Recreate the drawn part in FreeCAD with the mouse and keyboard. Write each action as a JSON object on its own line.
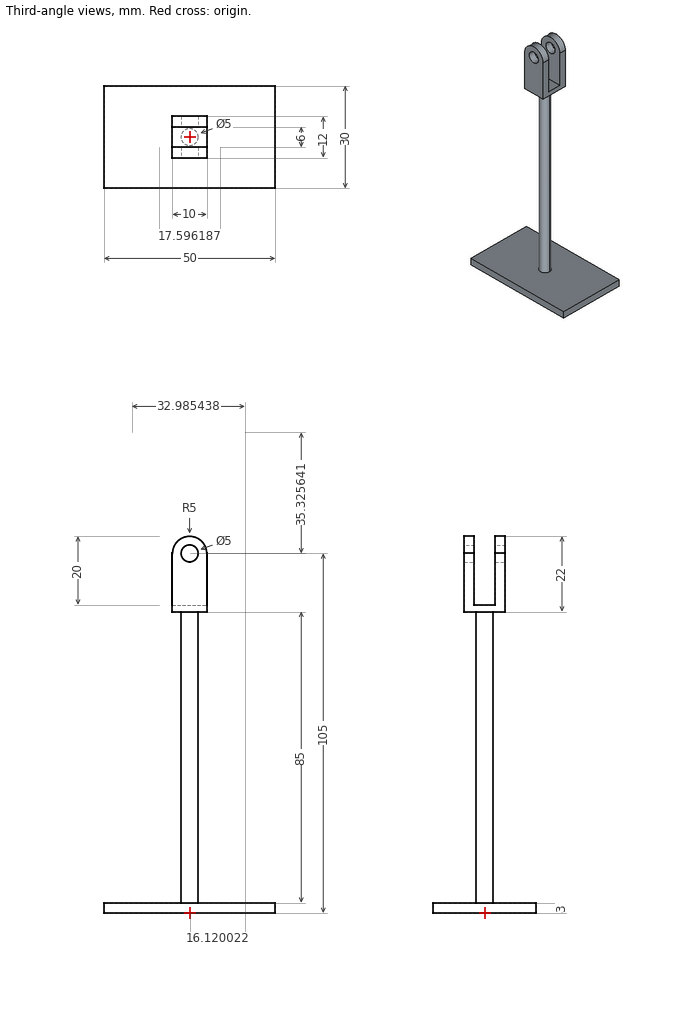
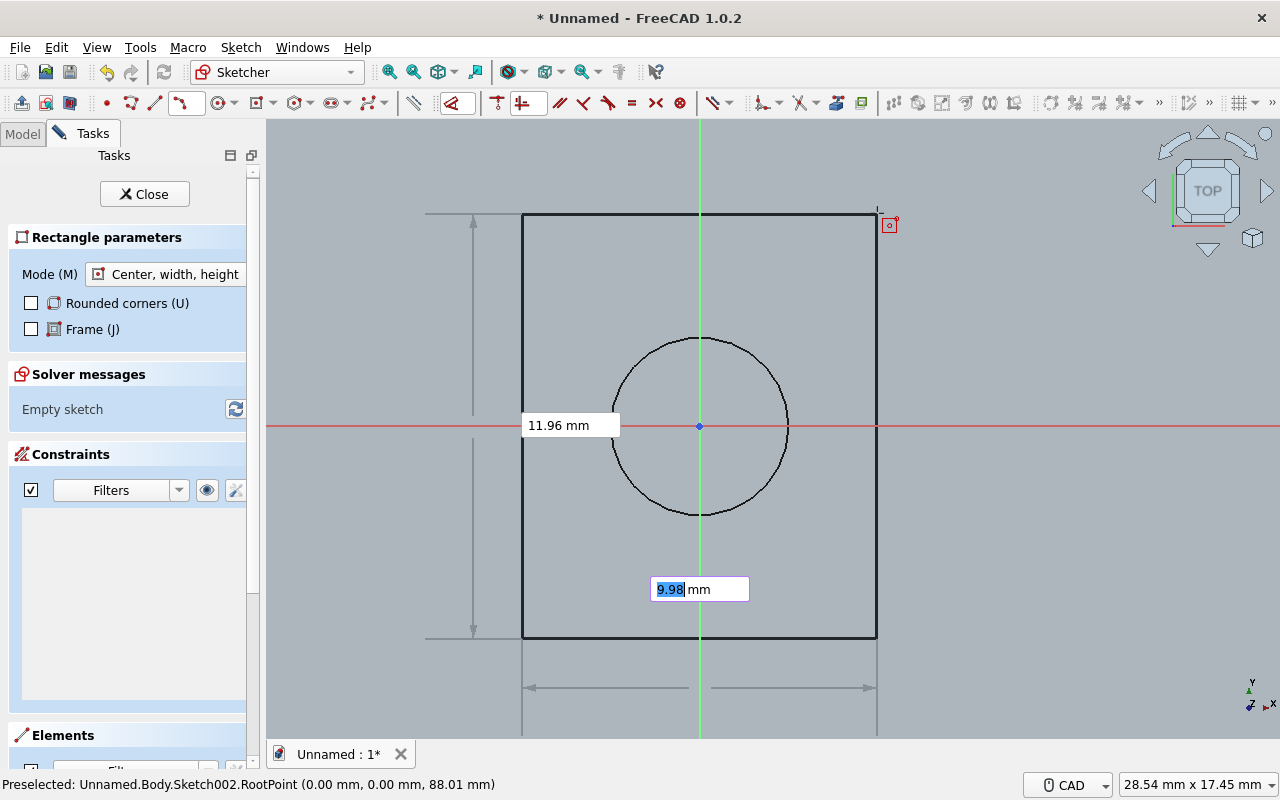
{"action": "type", "text": "10"}
{"action": "key", "text": "Tab"}
{"action": "type", "text": "12"}
{"action": "key", "text": "Return"}
{"action": "key", "text": "Escape"}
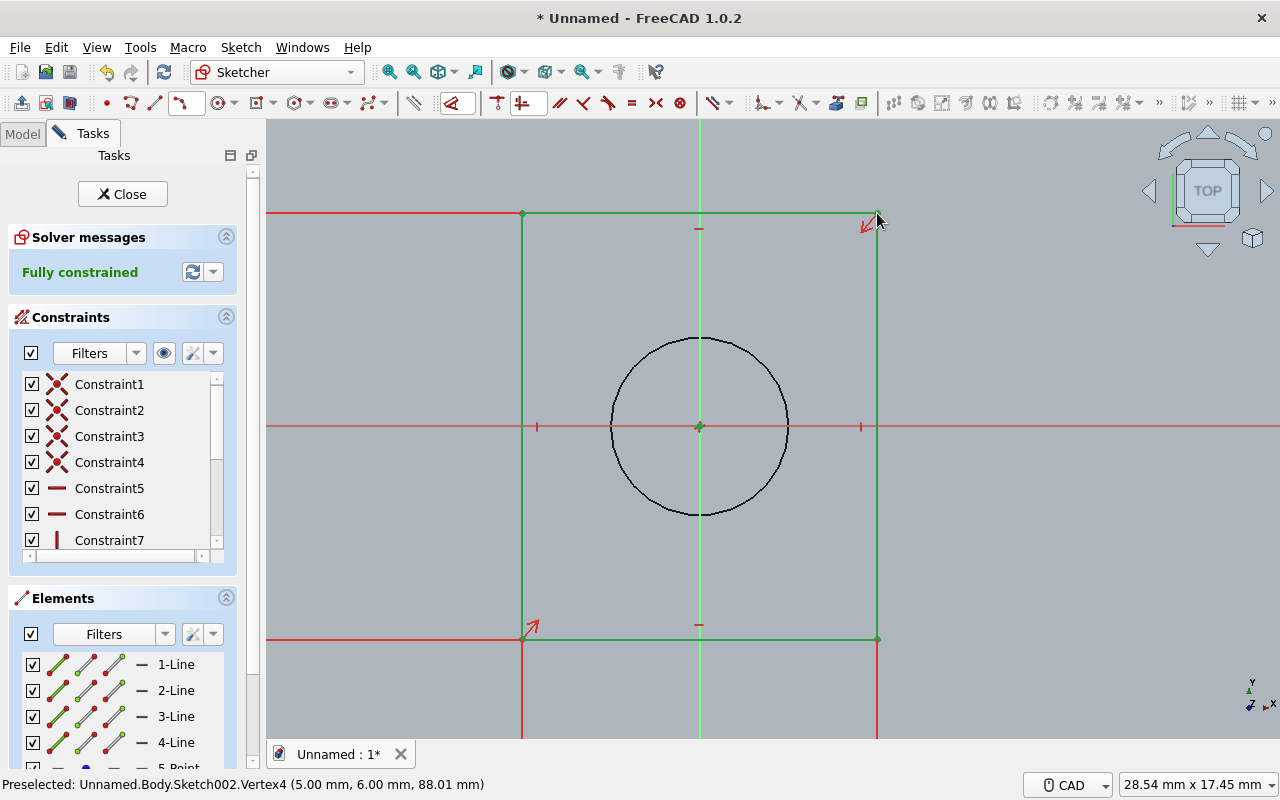
{"action": "left_click", "coordinate": [123, 194]}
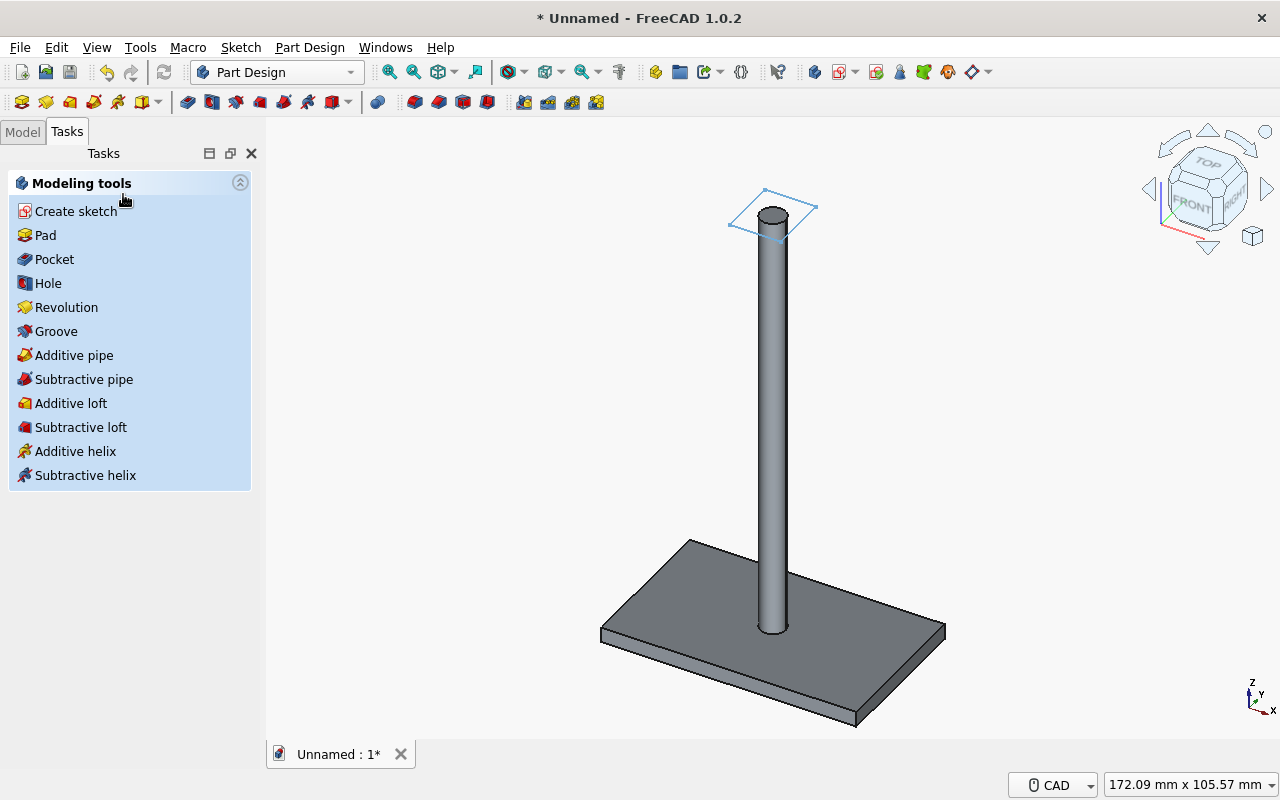
{"action": "left_click", "coordinate": [22, 102]}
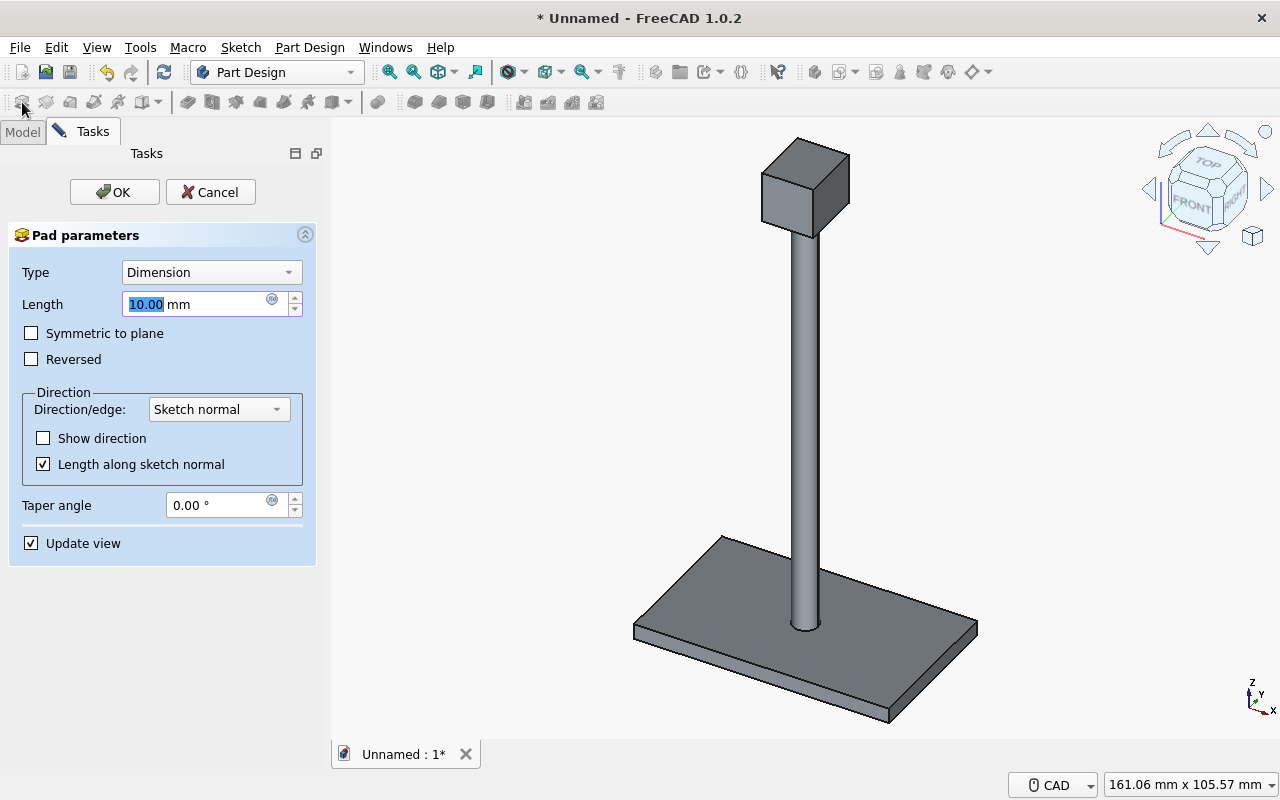
{"action": "type", "text": "22"}
{"action": "key", "text": "Tab"}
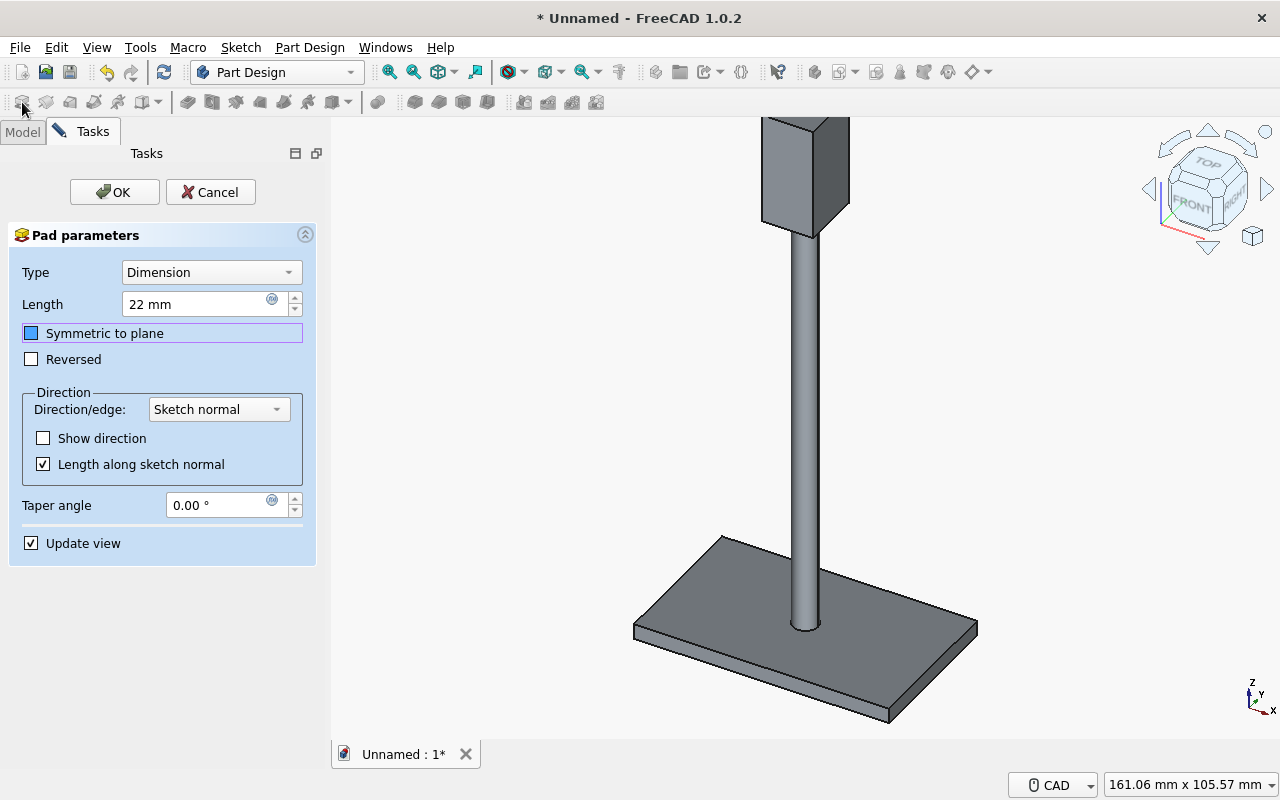
{"action": "left_click", "coordinate": [115, 192]}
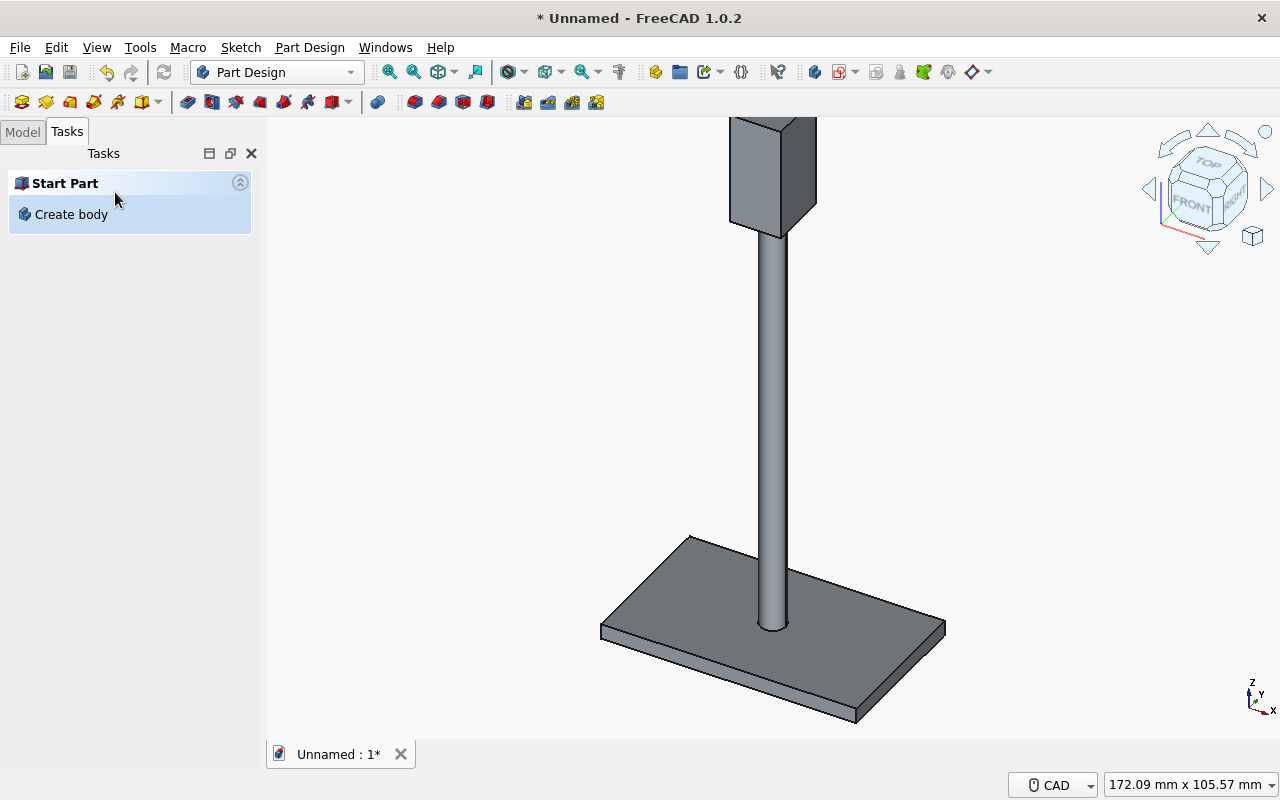
{"action": "left_click", "coordinate": [390, 72]}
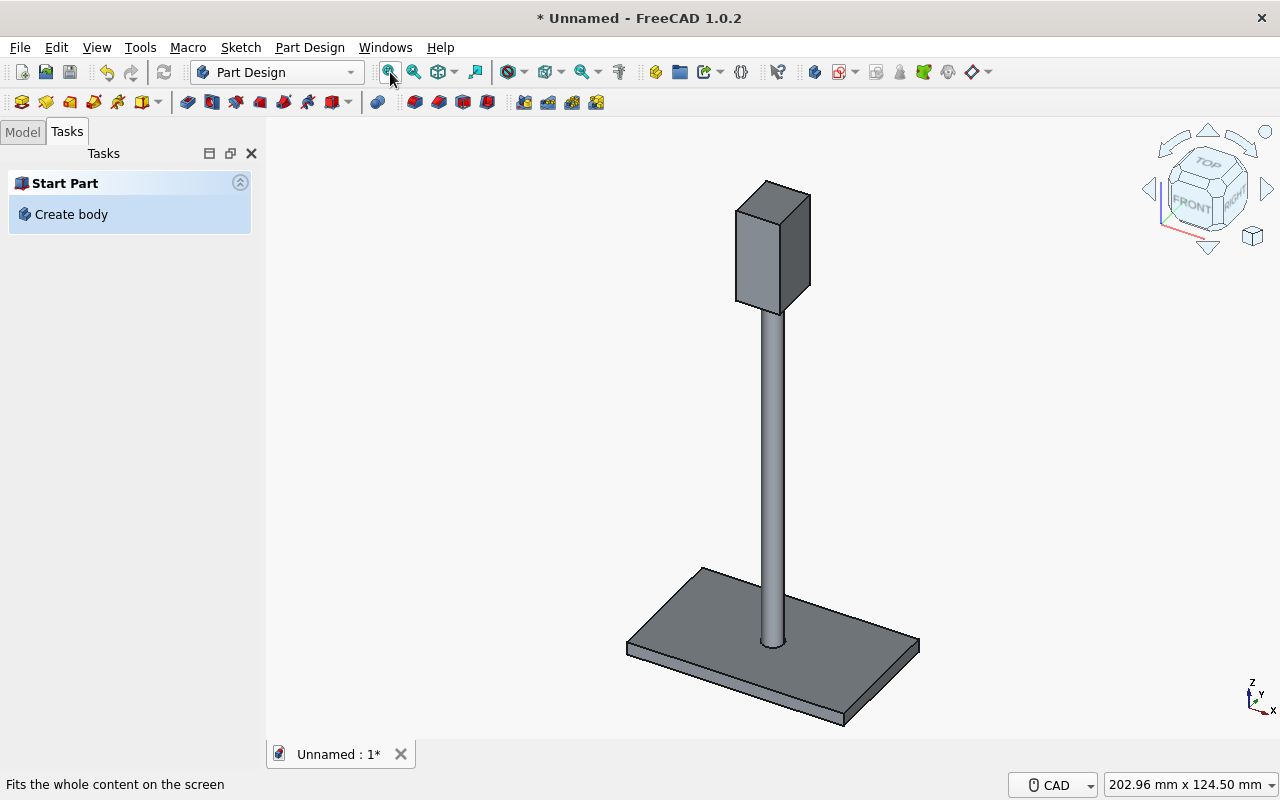
{"action": "left_click", "coordinate": [773, 202]}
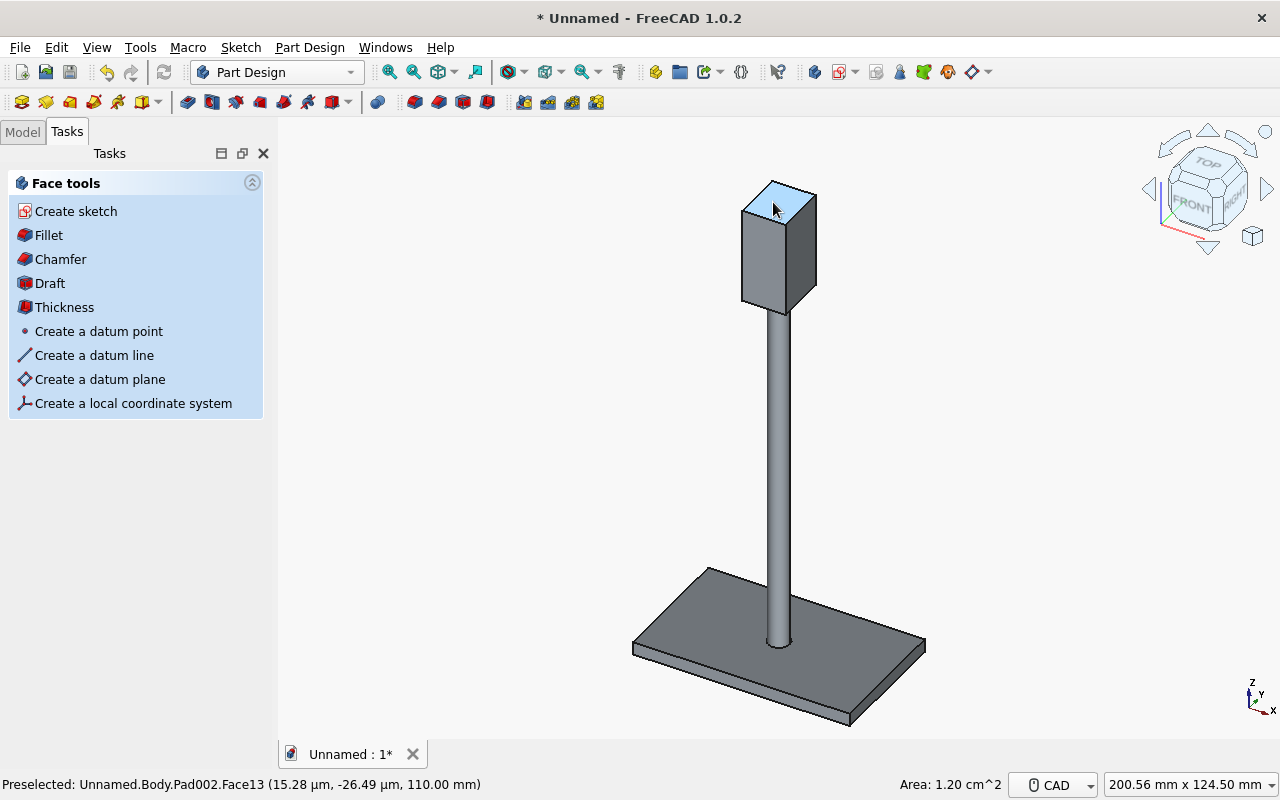
{"action": "left_click", "coordinate": [840, 72]}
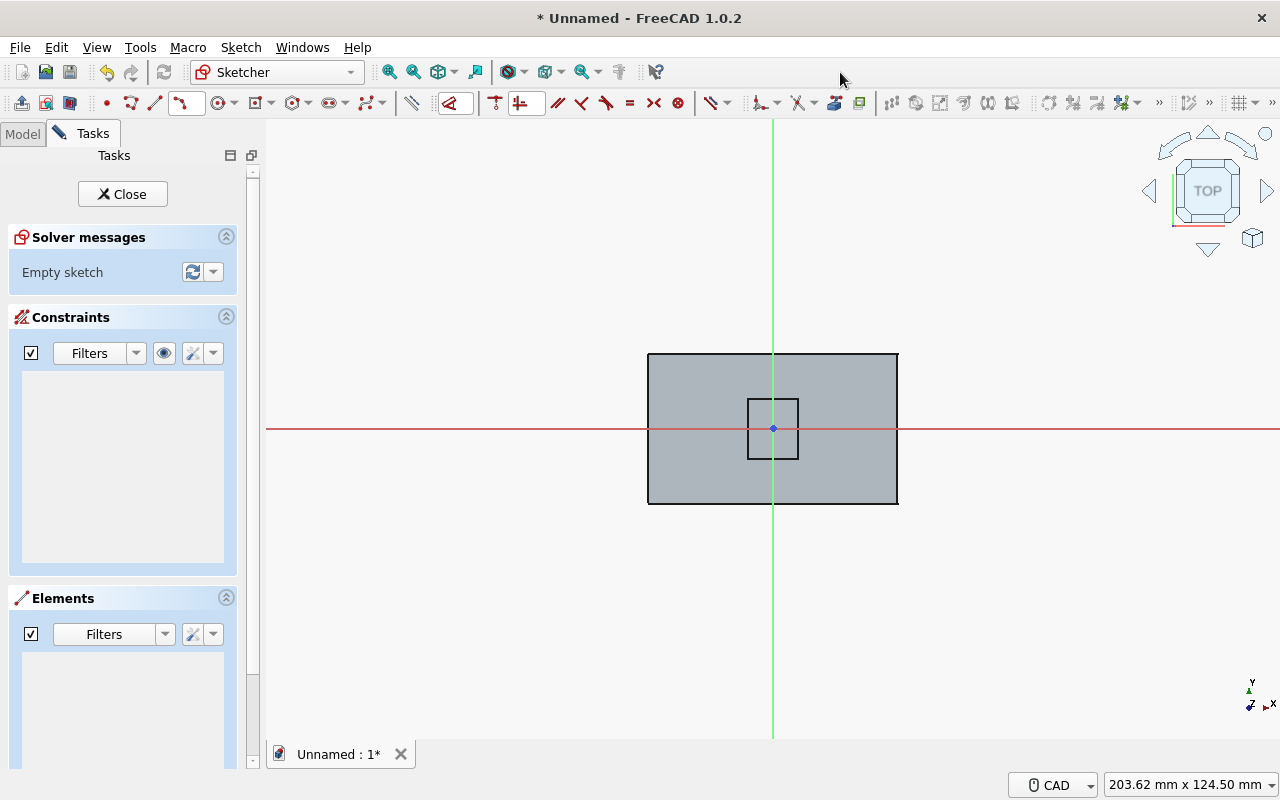
{"action": "scroll", "coordinate": [787, 429], "scroll_direction": "up", "scroll_amount": 9}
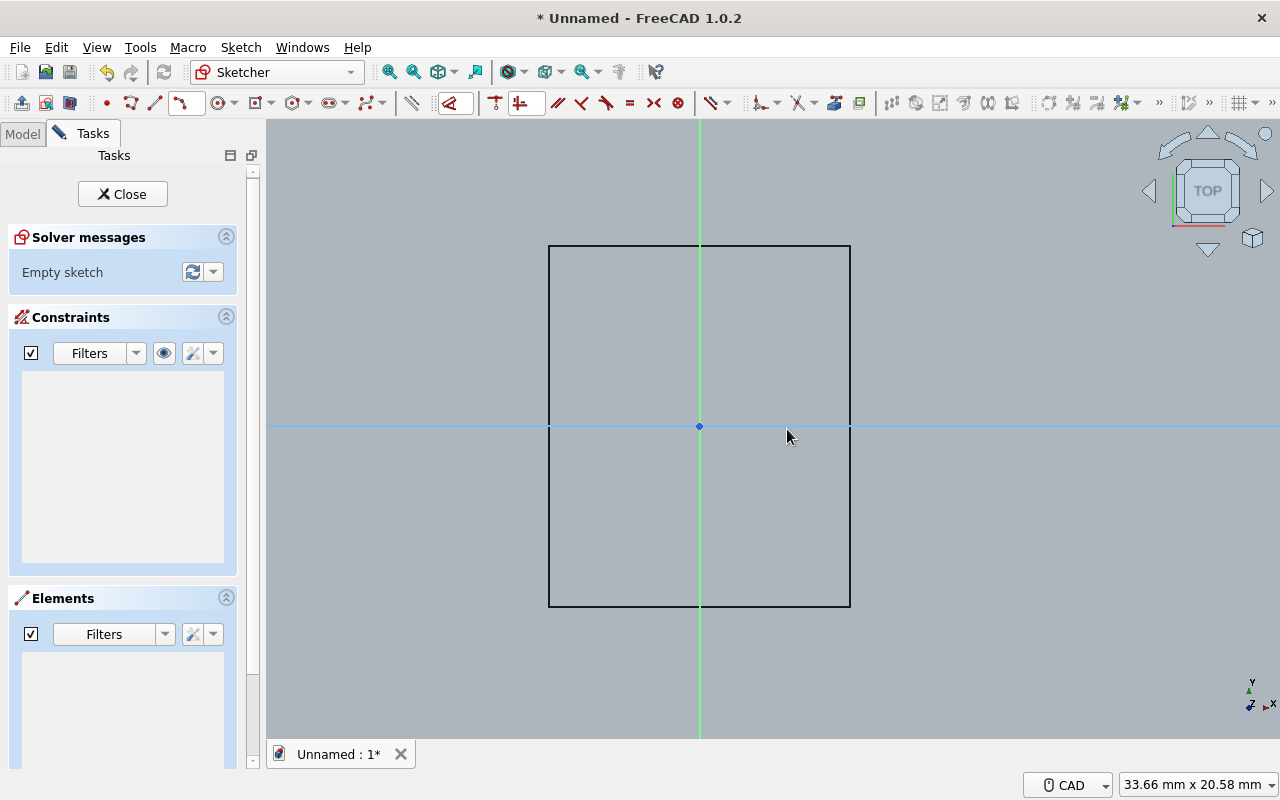
{"action": "left_click", "coordinate": [256, 104]}